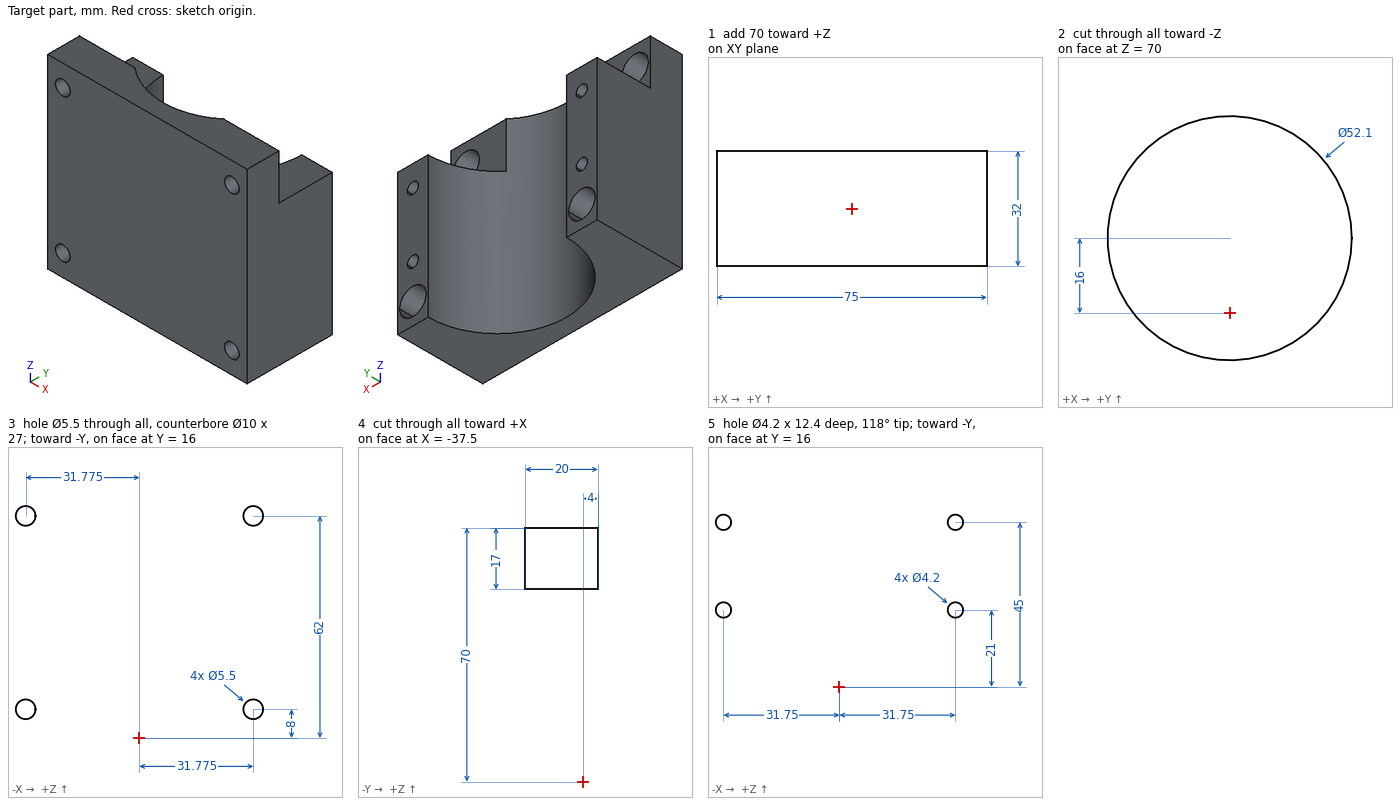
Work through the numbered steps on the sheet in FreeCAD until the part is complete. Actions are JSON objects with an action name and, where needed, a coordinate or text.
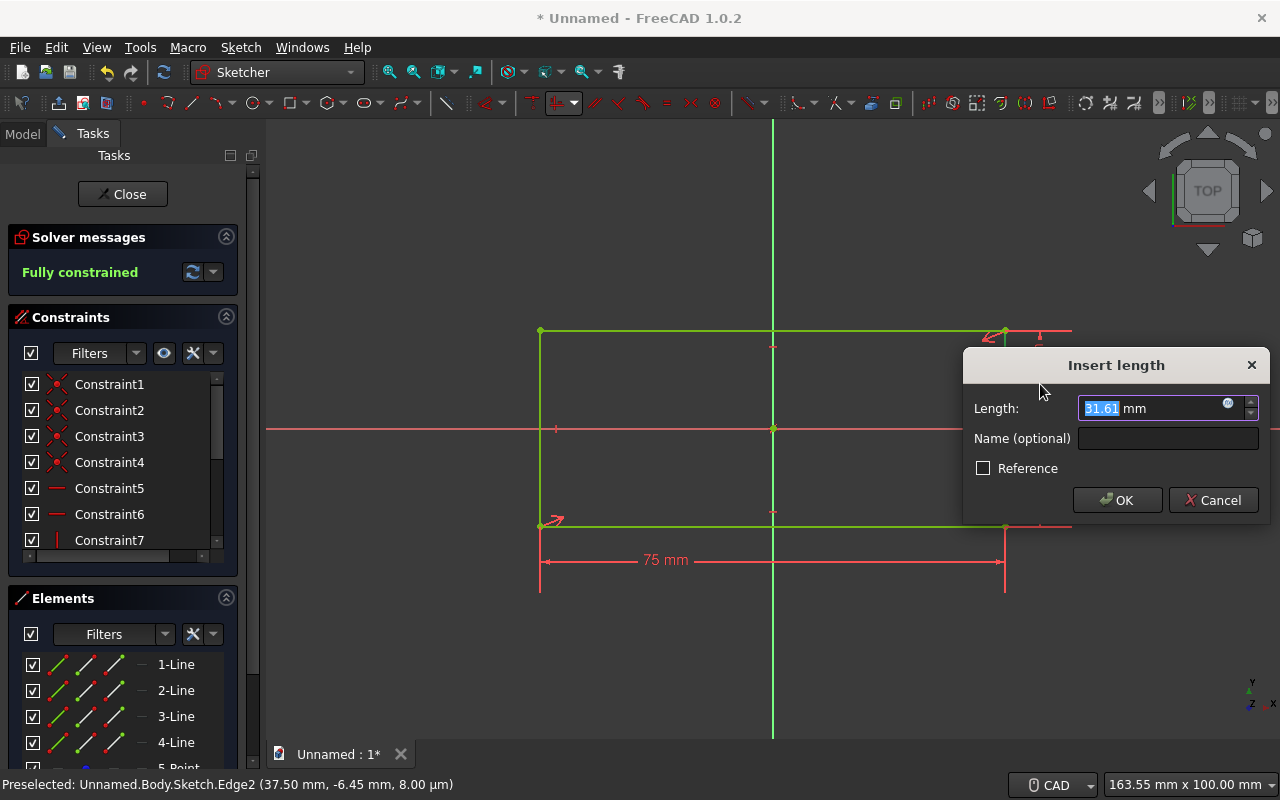
{"action": "type", "text": "32"}
{"action": "key", "text": "Return"}
{"action": "key", "text": "Escape"}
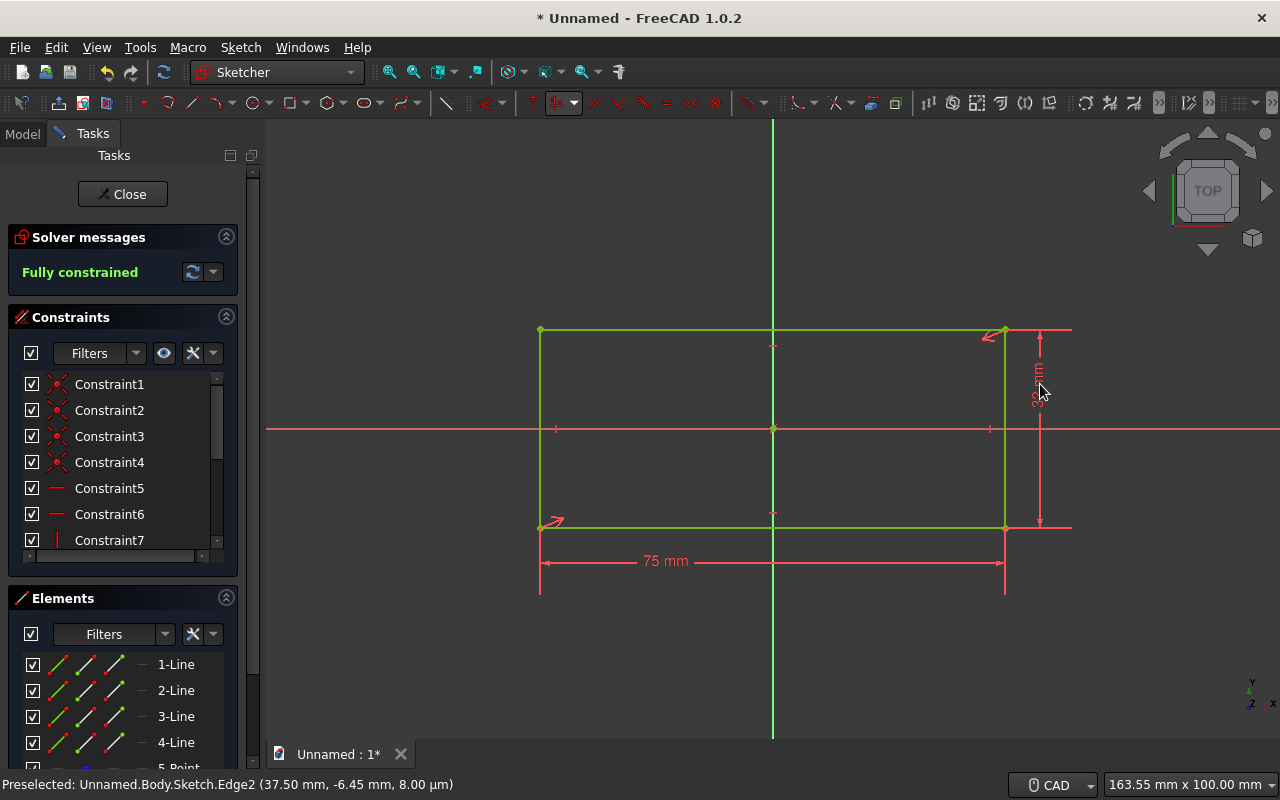
{"action": "left_click", "coordinate": [123, 194]}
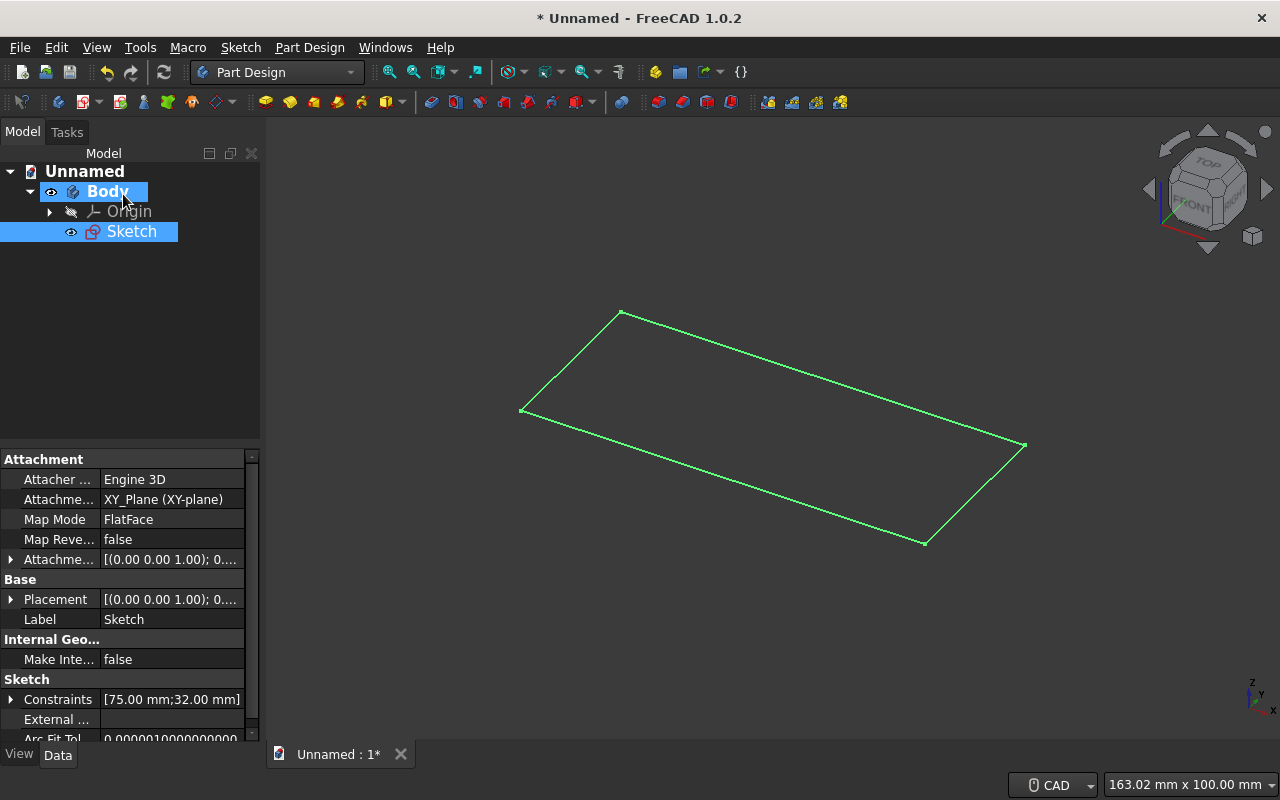
{"action": "left_click", "coordinate": [266, 102]}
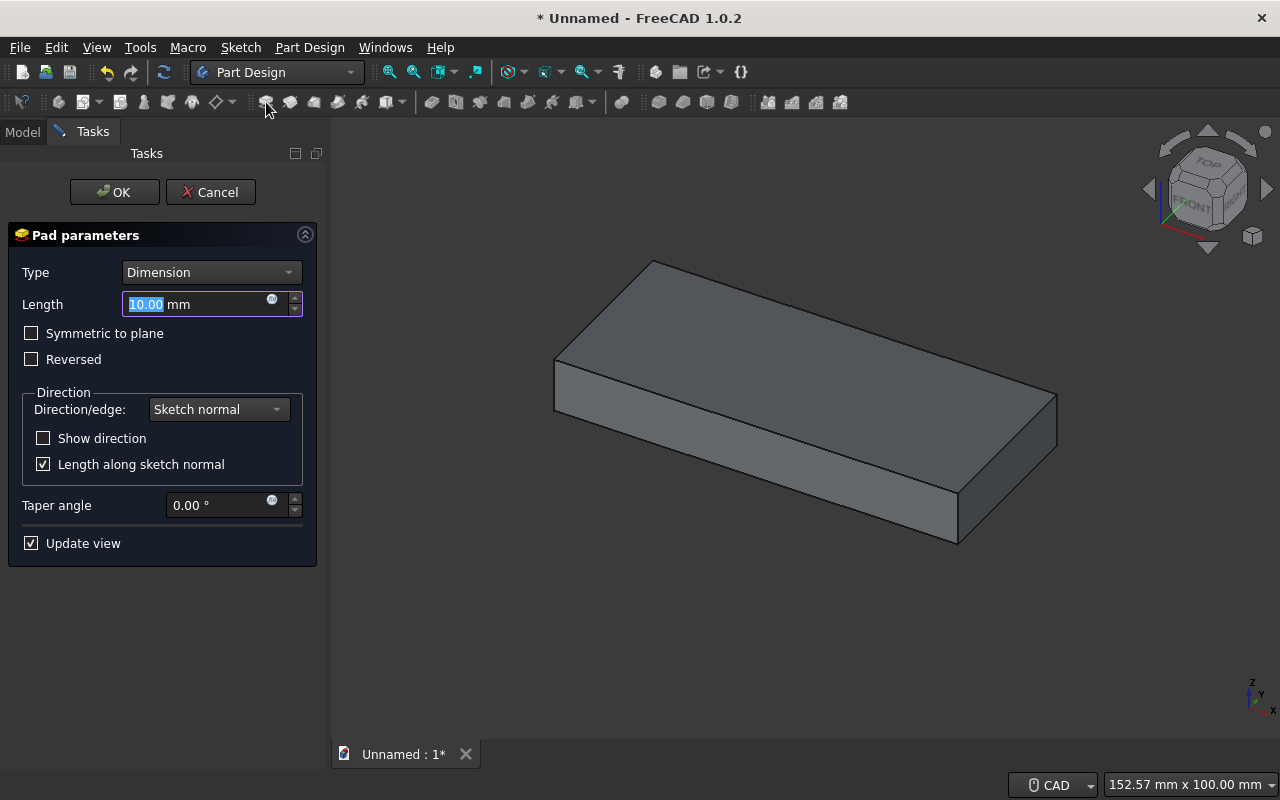
{"action": "type", "text": "70"}
{"action": "key", "text": "Tab"}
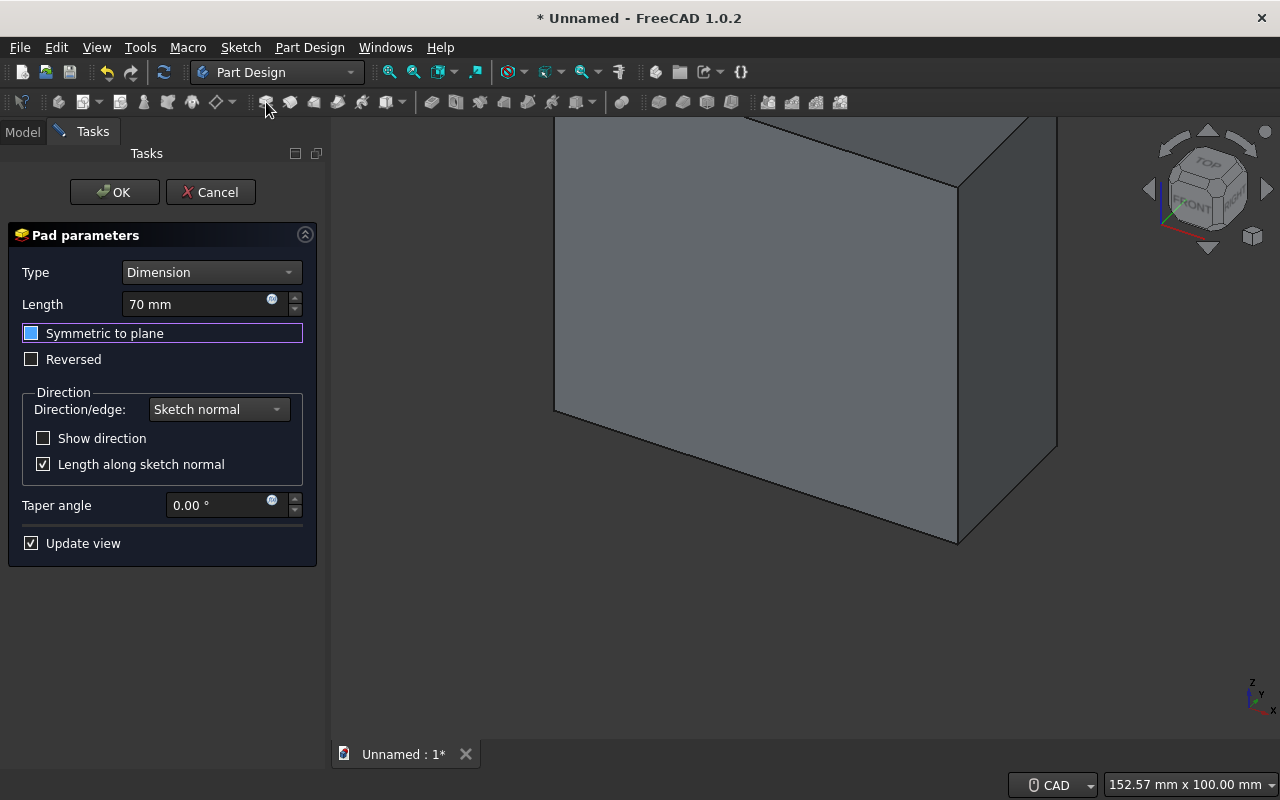
{"action": "left_click", "coordinate": [115, 192]}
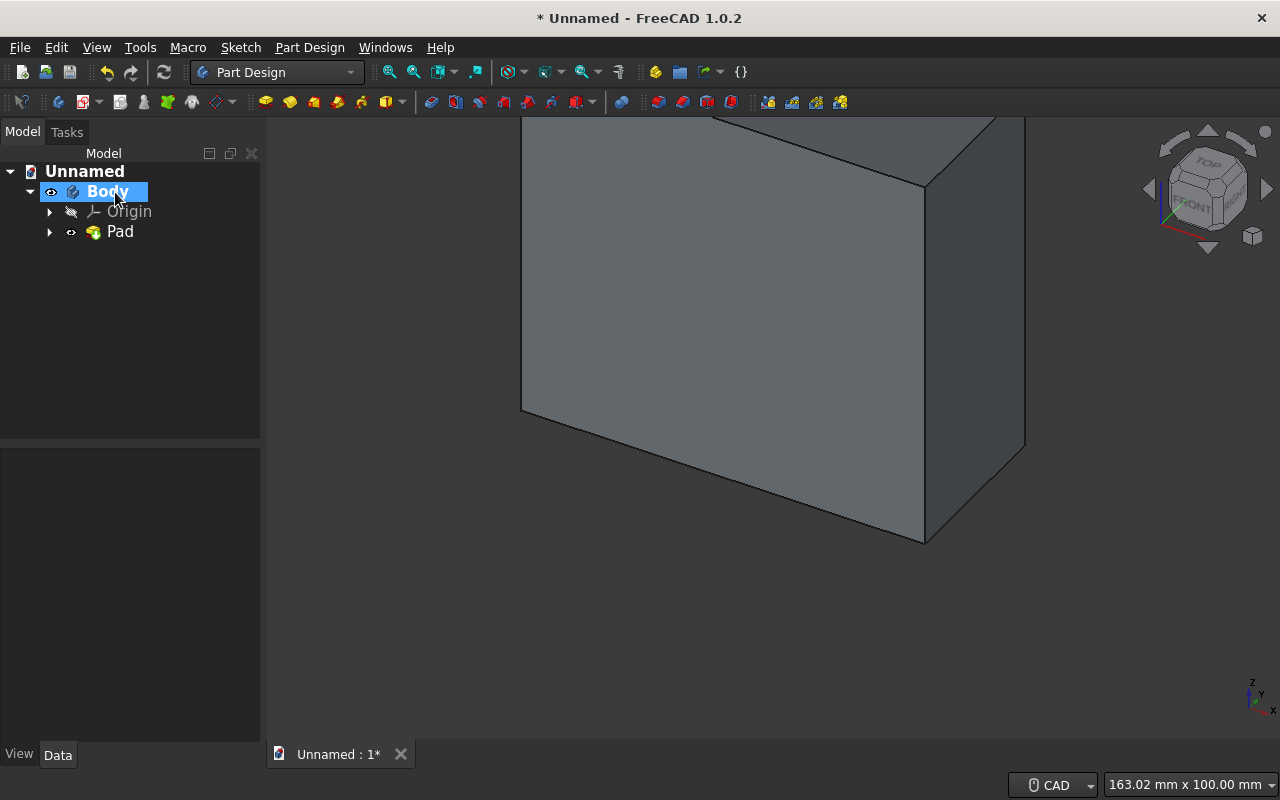
{"action": "left_click", "coordinate": [390, 72]}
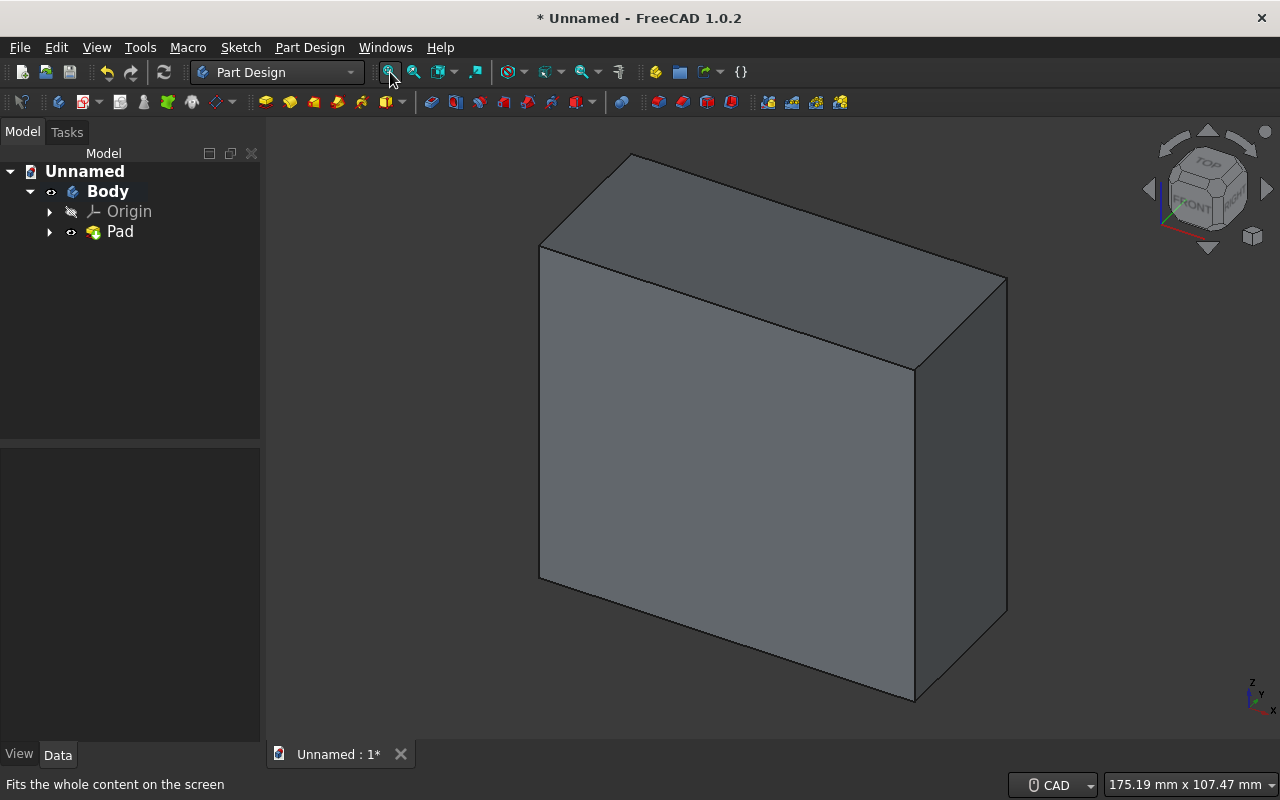
{"action": "left_click", "coordinate": [880, 297]}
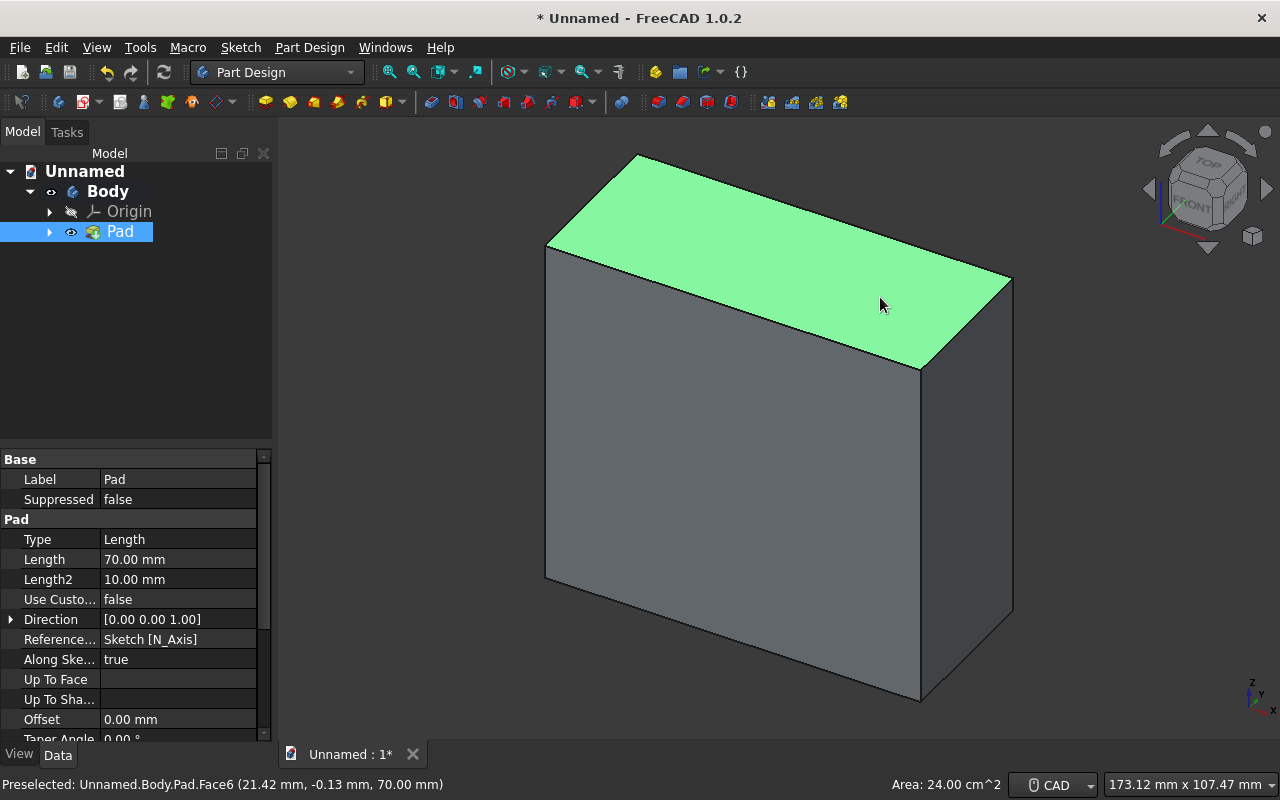
{"action": "left_click", "coordinate": [84, 102]}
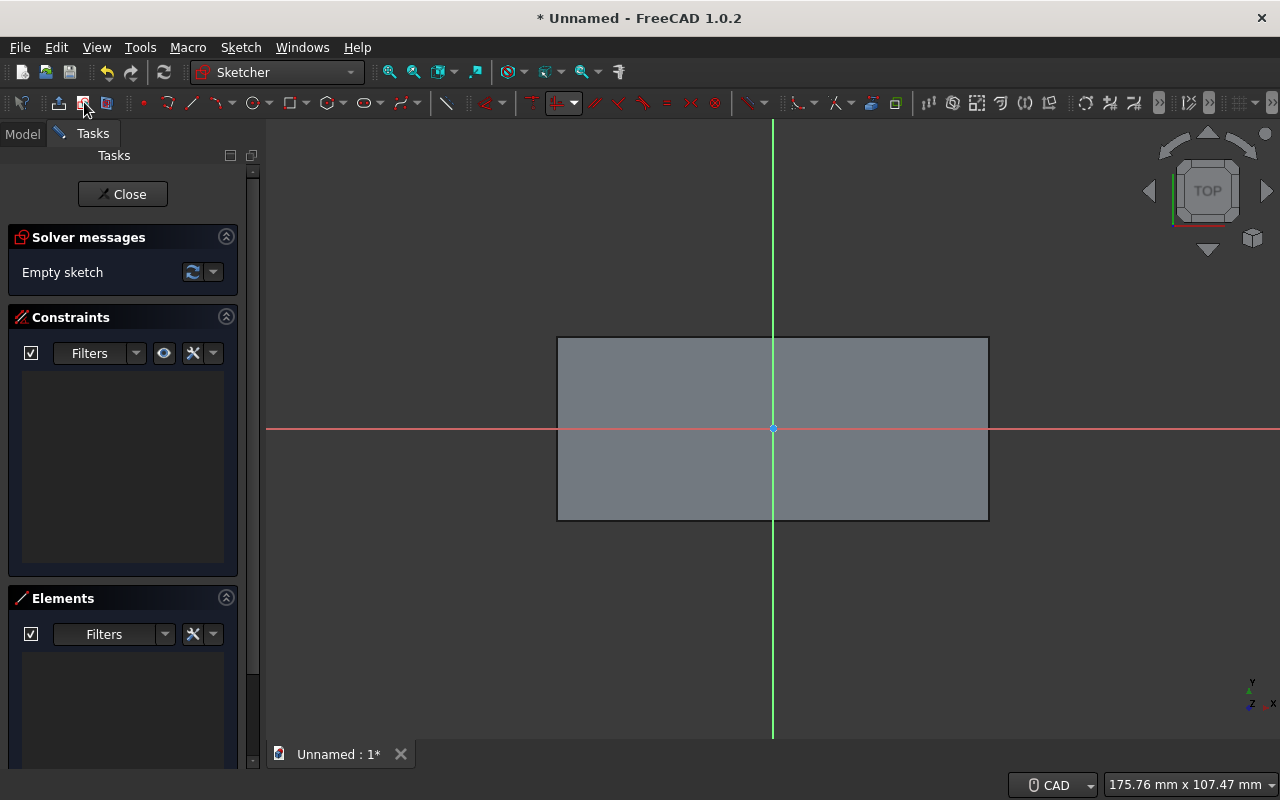
{"action": "left_click", "coordinate": [254, 104]}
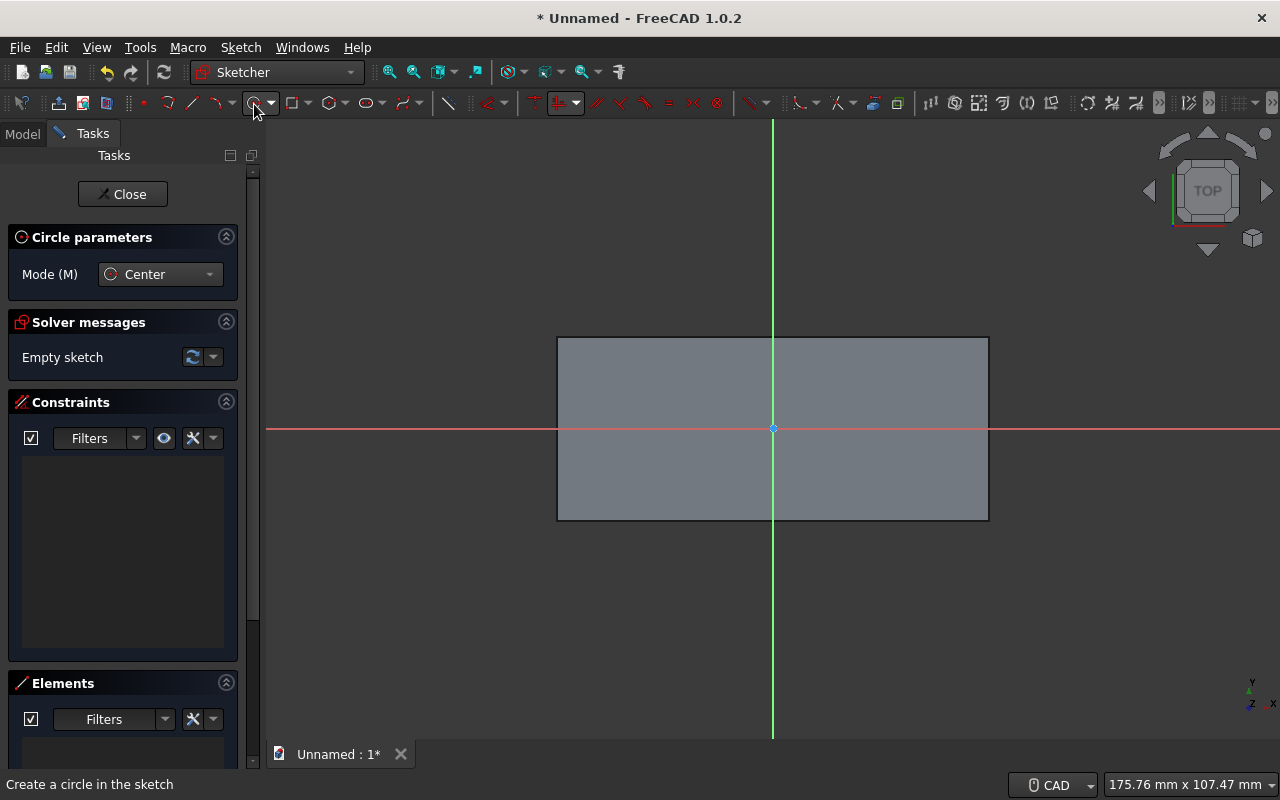
{"action": "left_click", "coordinate": [773, 337]}
{"action": "left_click", "coordinate": [879, 230]}
{"action": "key", "text": "Escape"}